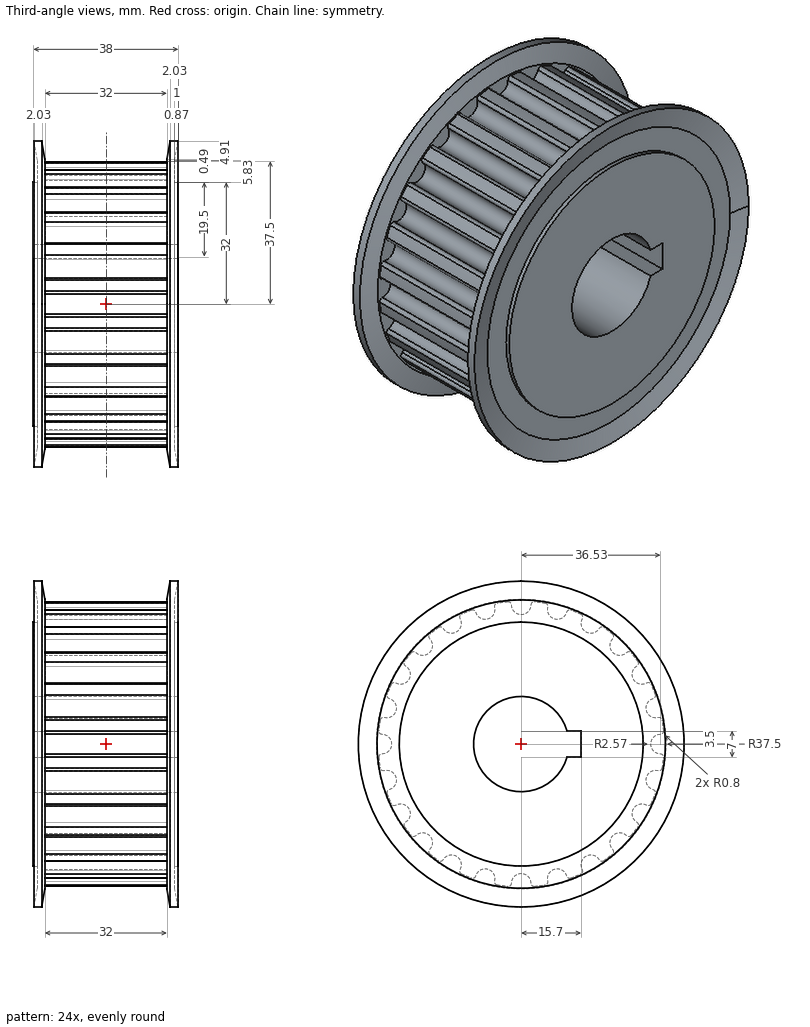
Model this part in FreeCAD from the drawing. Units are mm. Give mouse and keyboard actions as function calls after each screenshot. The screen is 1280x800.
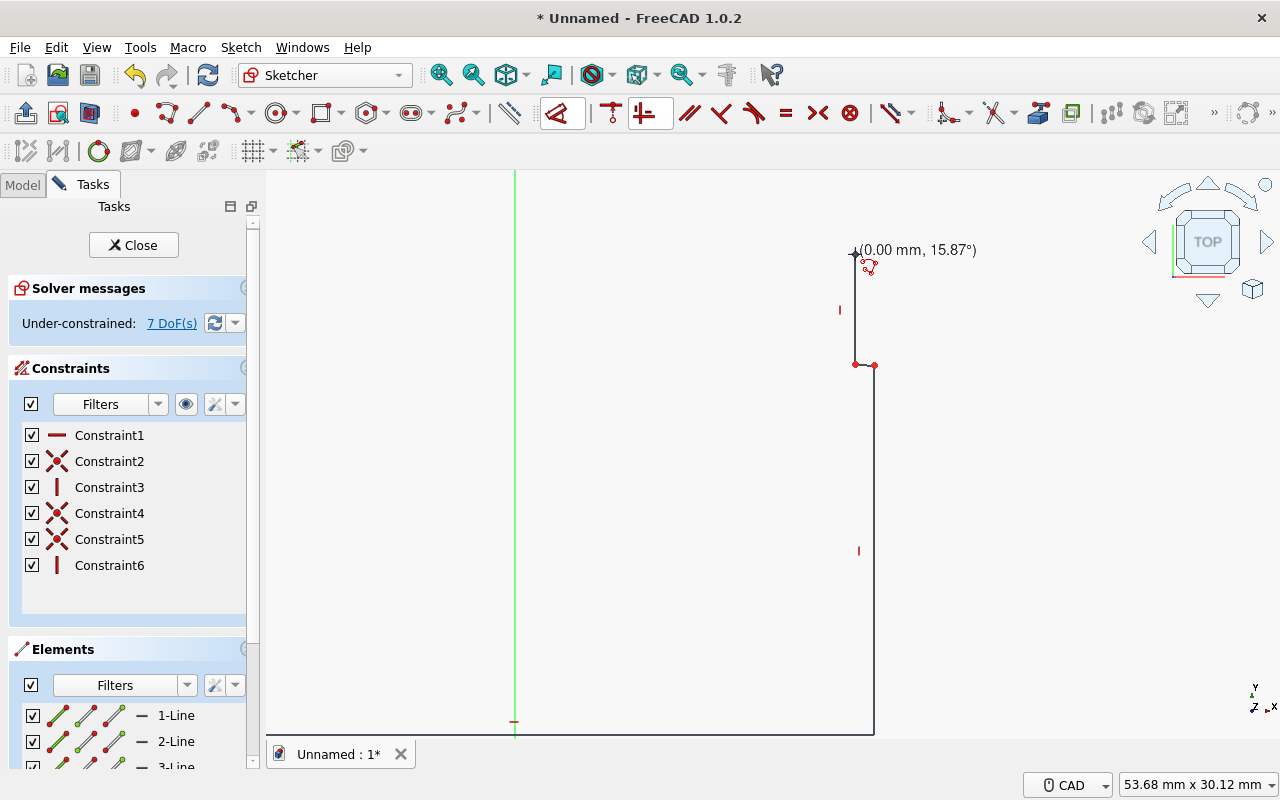
scroll(859, 364, down, 4)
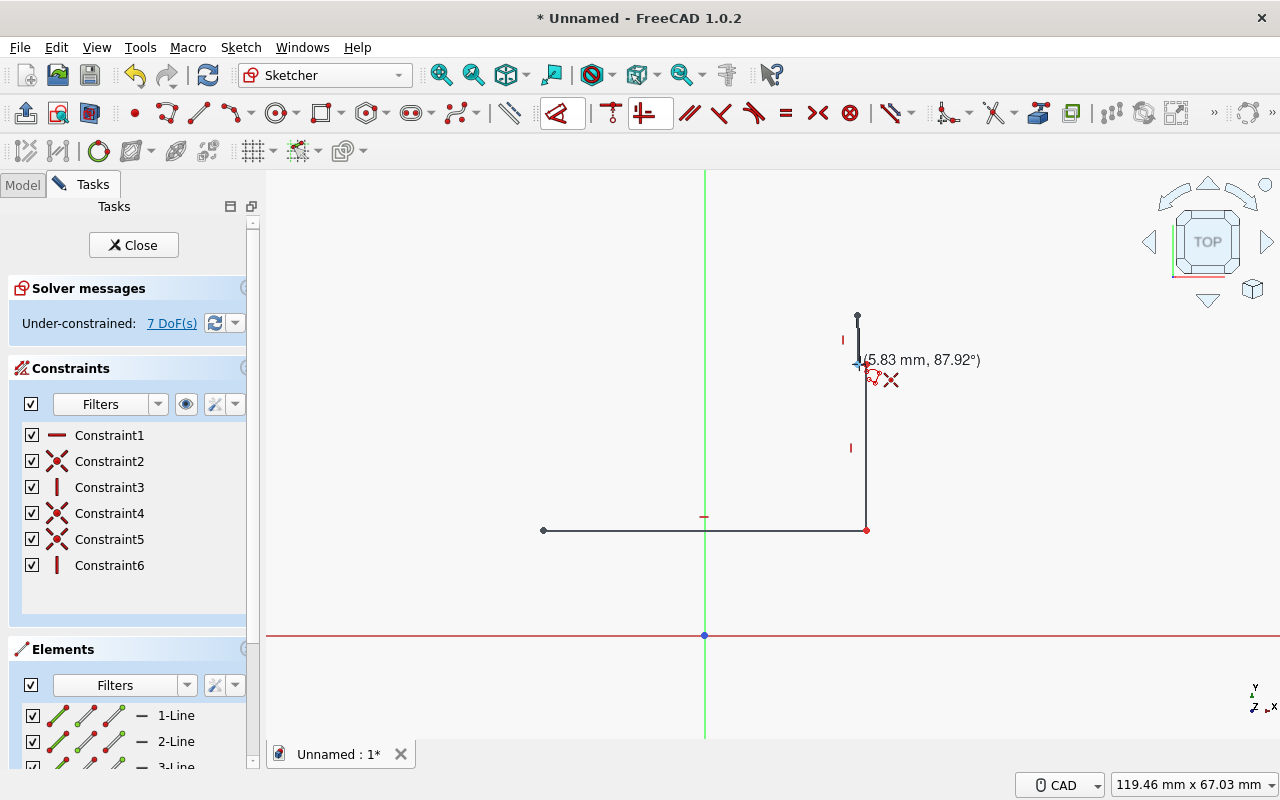
click(865, 273)
click(848, 273)
click(841, 313)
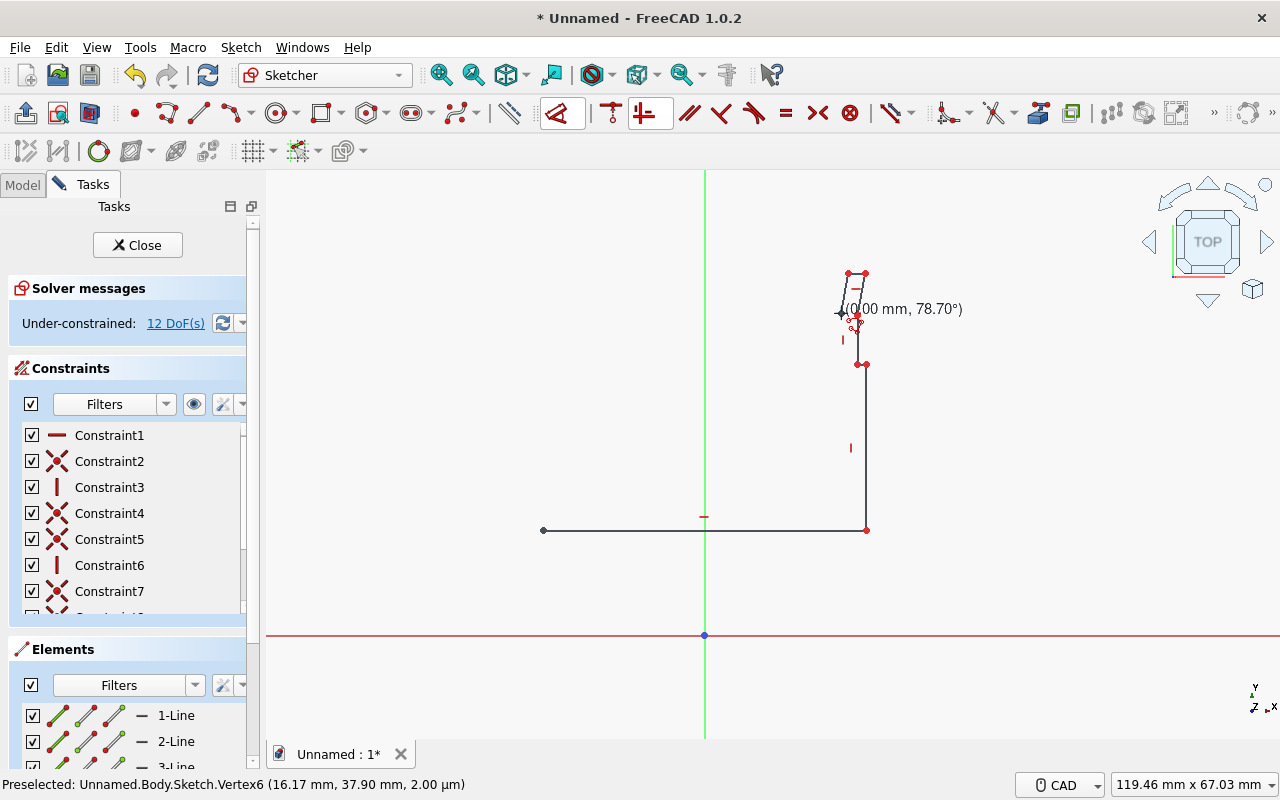
scroll(841, 318, up, 7)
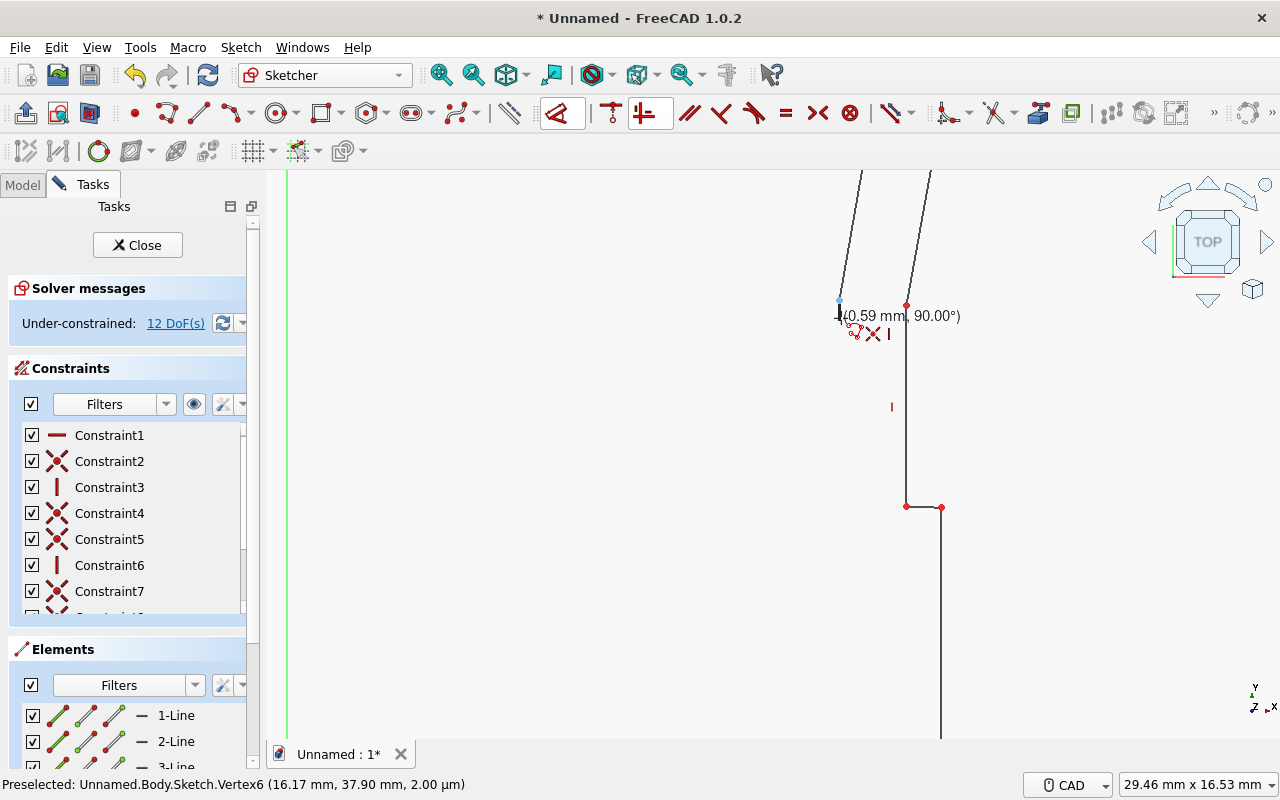
click(839, 315)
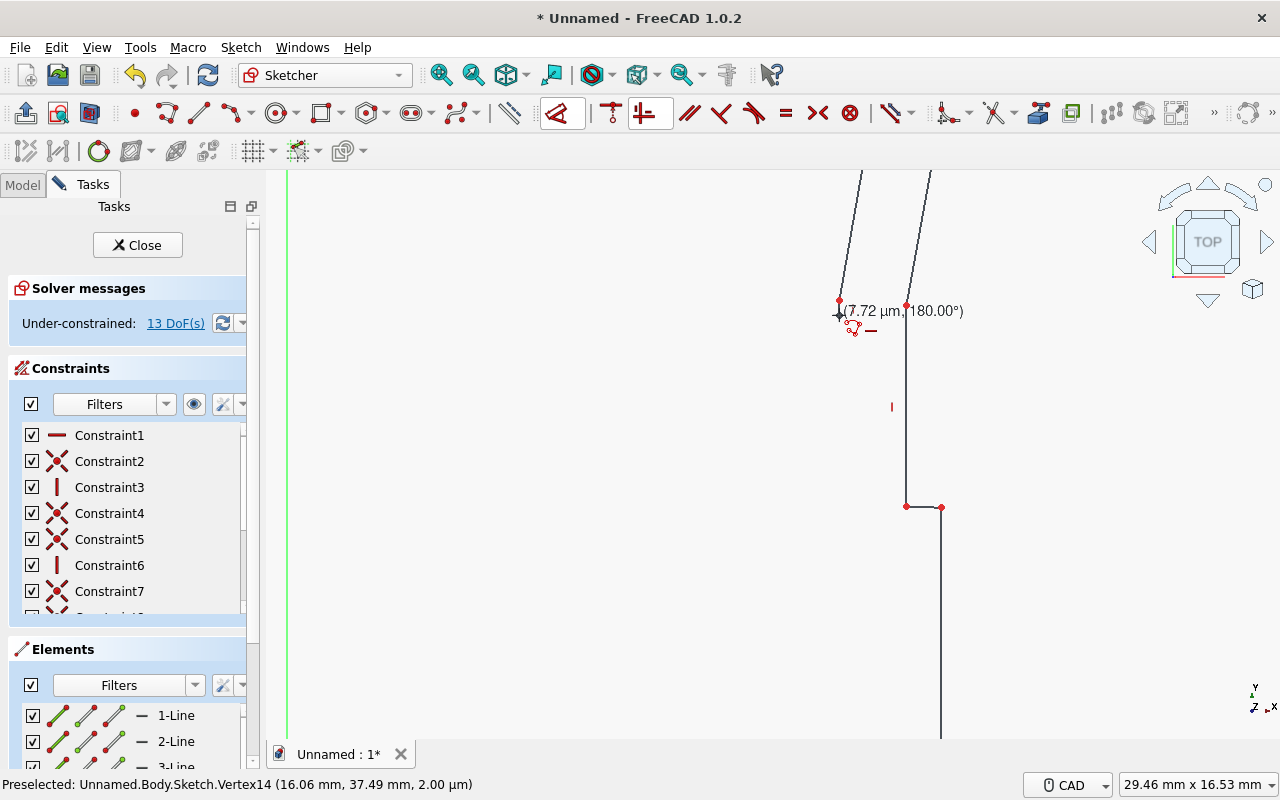
scroll(841, 318, down, 7)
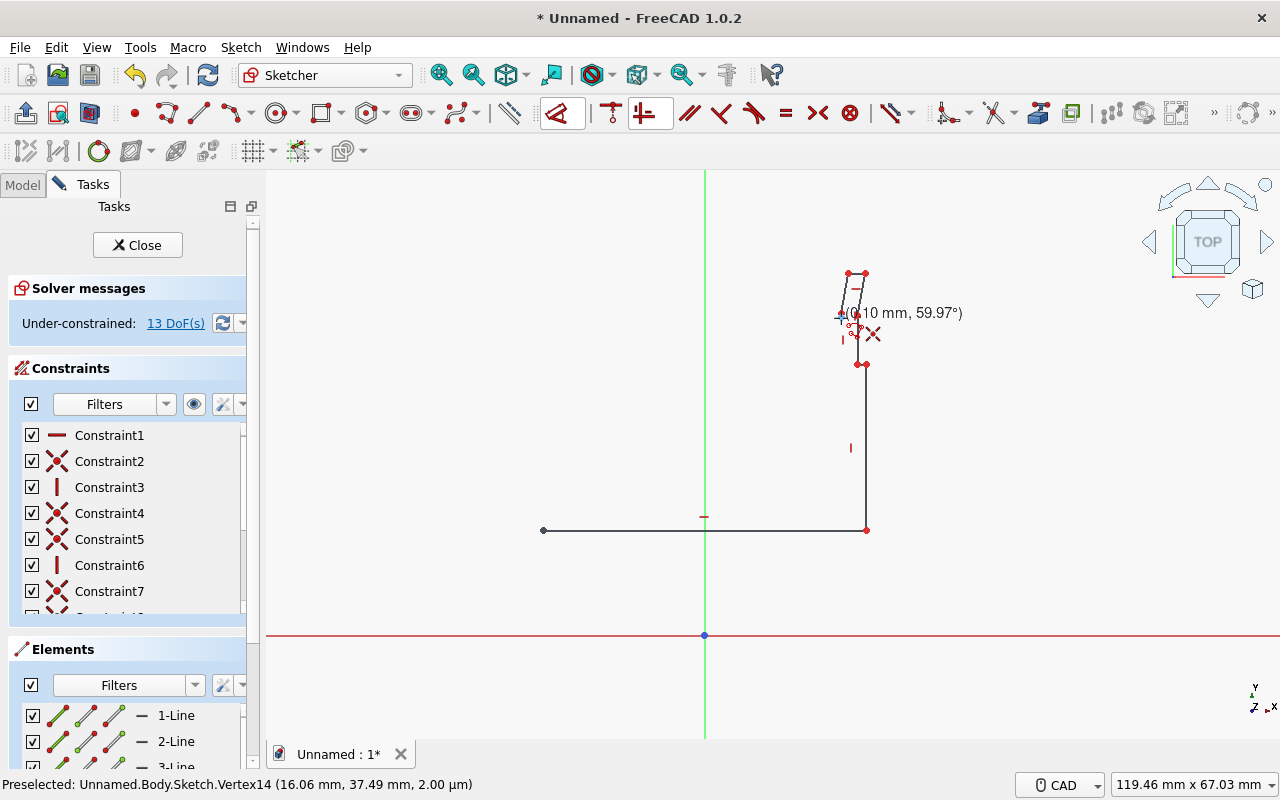
click(569, 317)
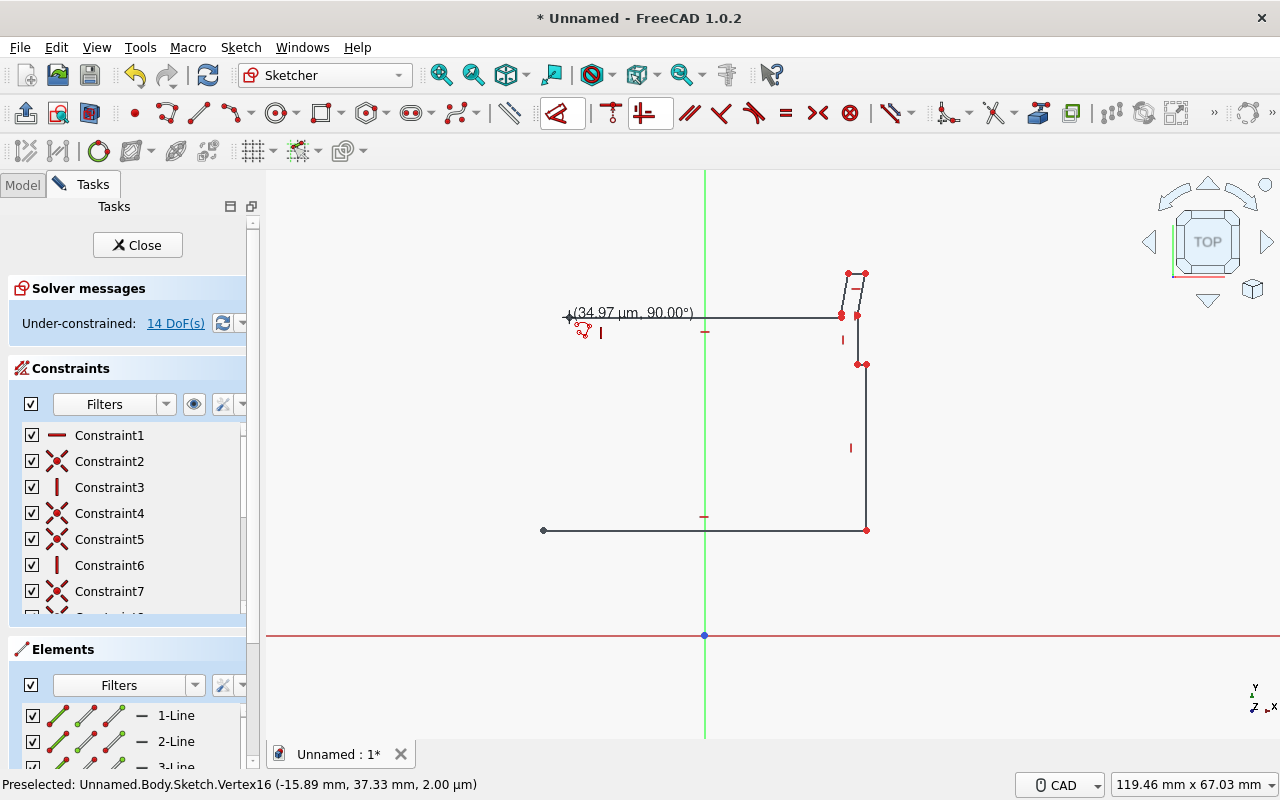
scroll(569, 313, up, 7)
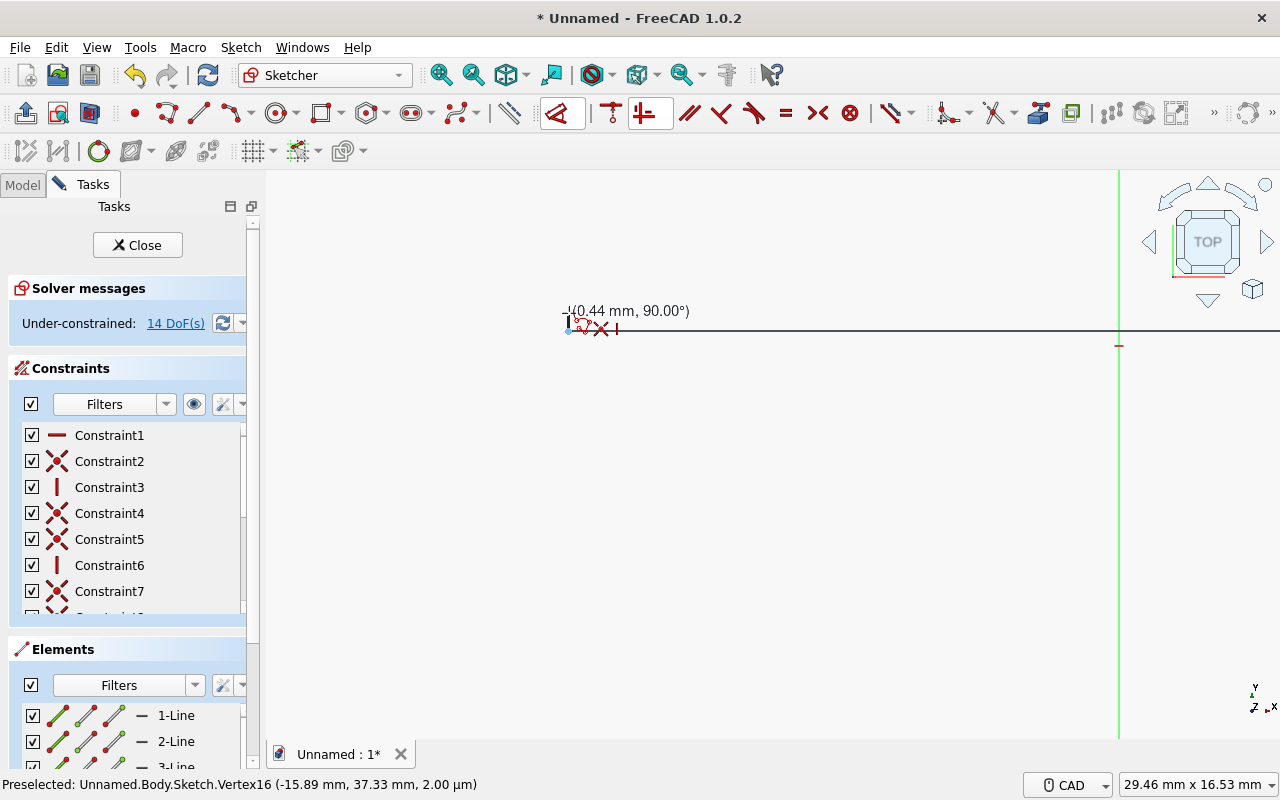
click(568, 314)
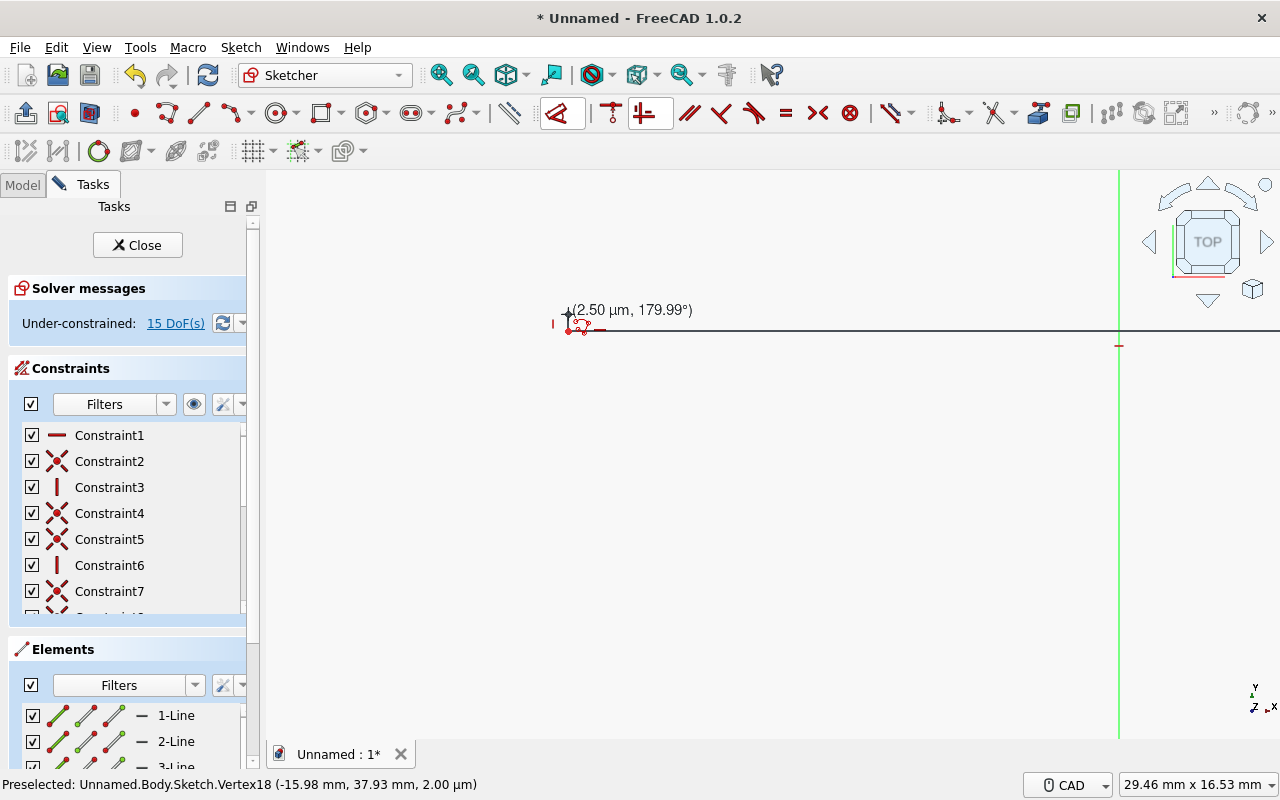
scroll(569, 313, down, 7)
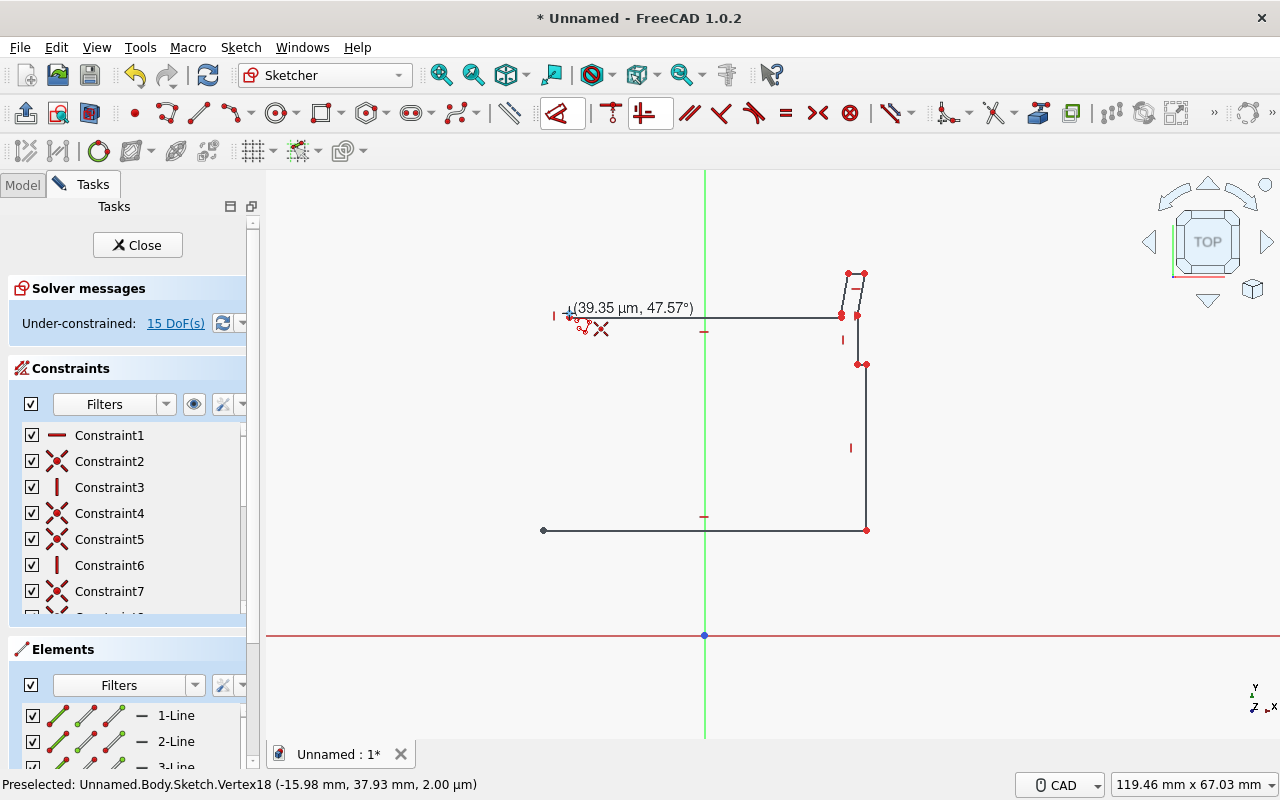
click(562, 273)
click(545, 273)
click(552, 315)
click(552, 364)